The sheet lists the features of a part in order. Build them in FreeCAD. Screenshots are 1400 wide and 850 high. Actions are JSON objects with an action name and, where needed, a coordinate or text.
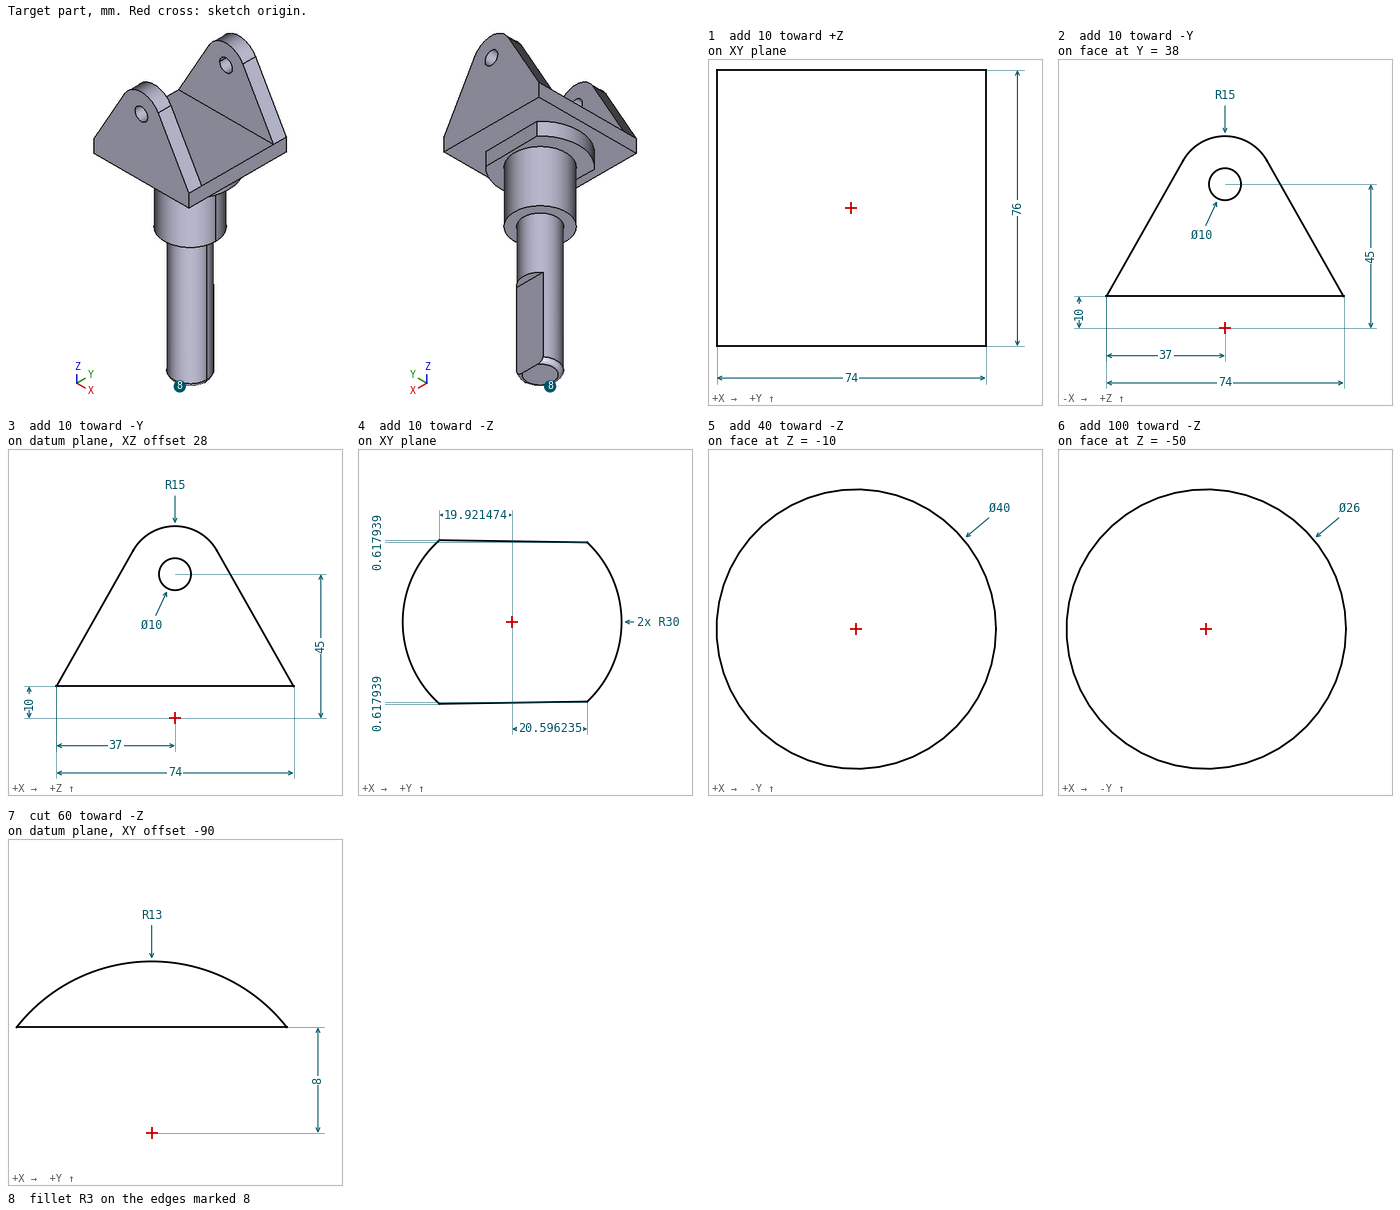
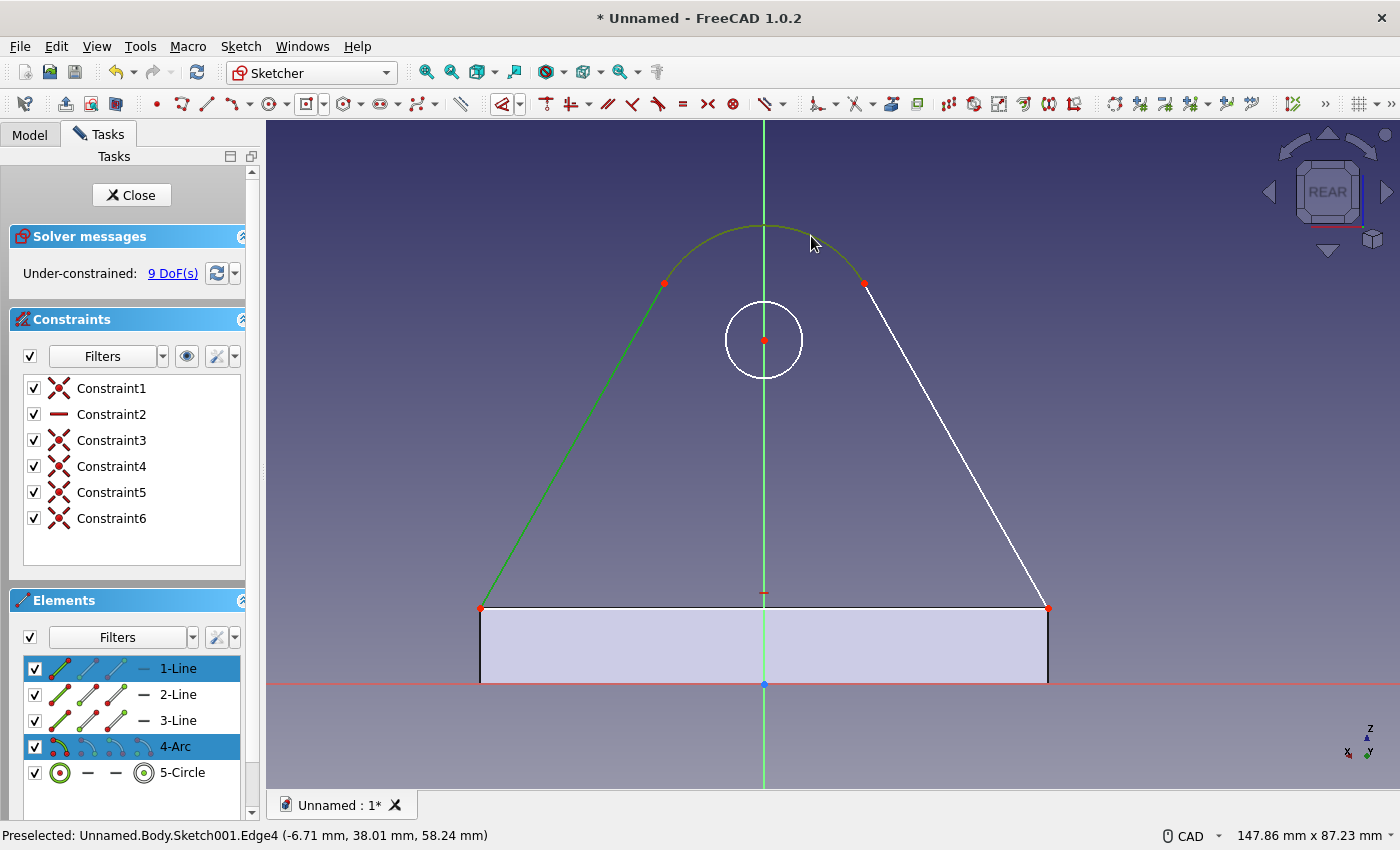
{"action": "left_click", "coordinate": [658, 104]}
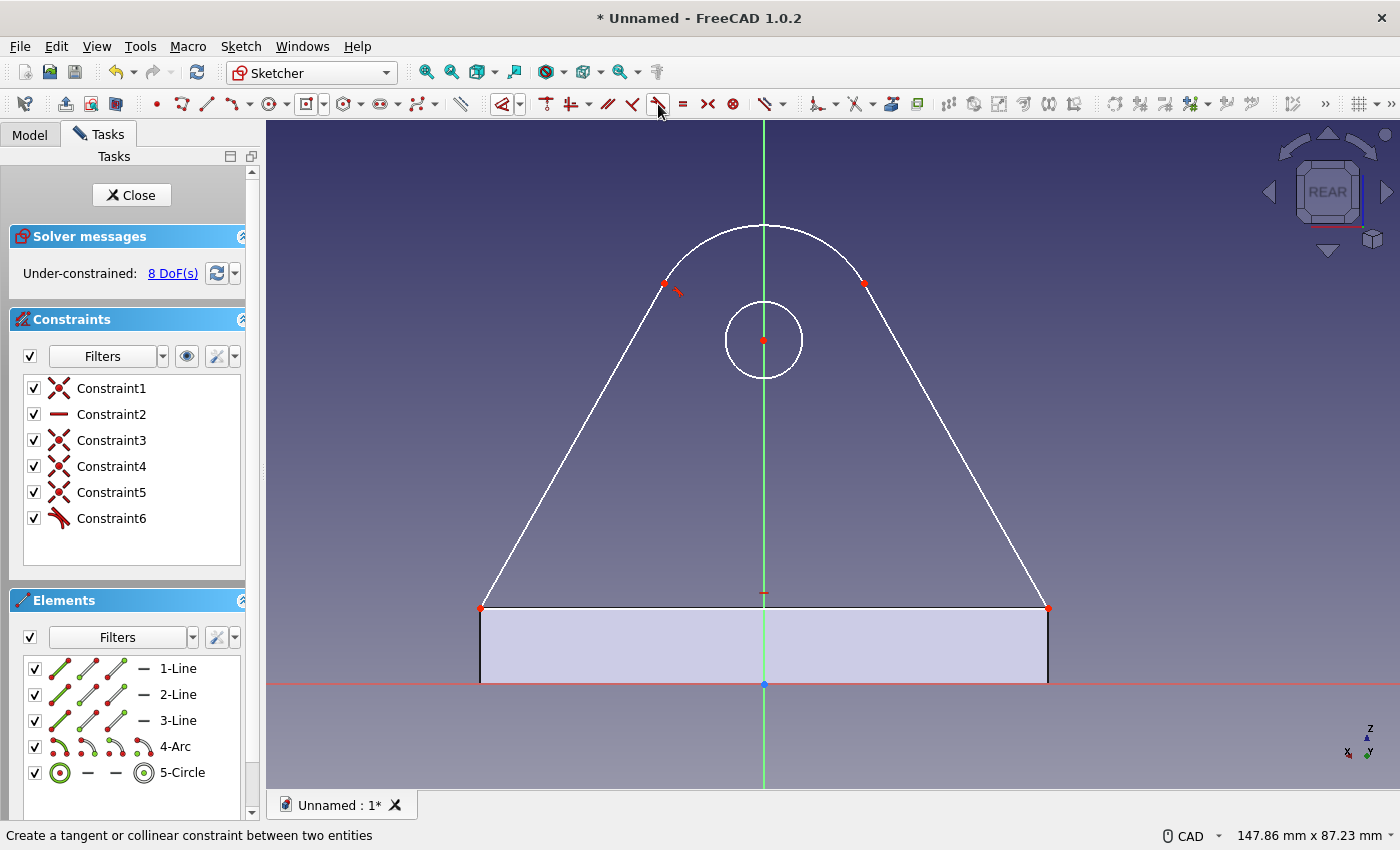
{"action": "left_click", "coordinate": [993, 511]}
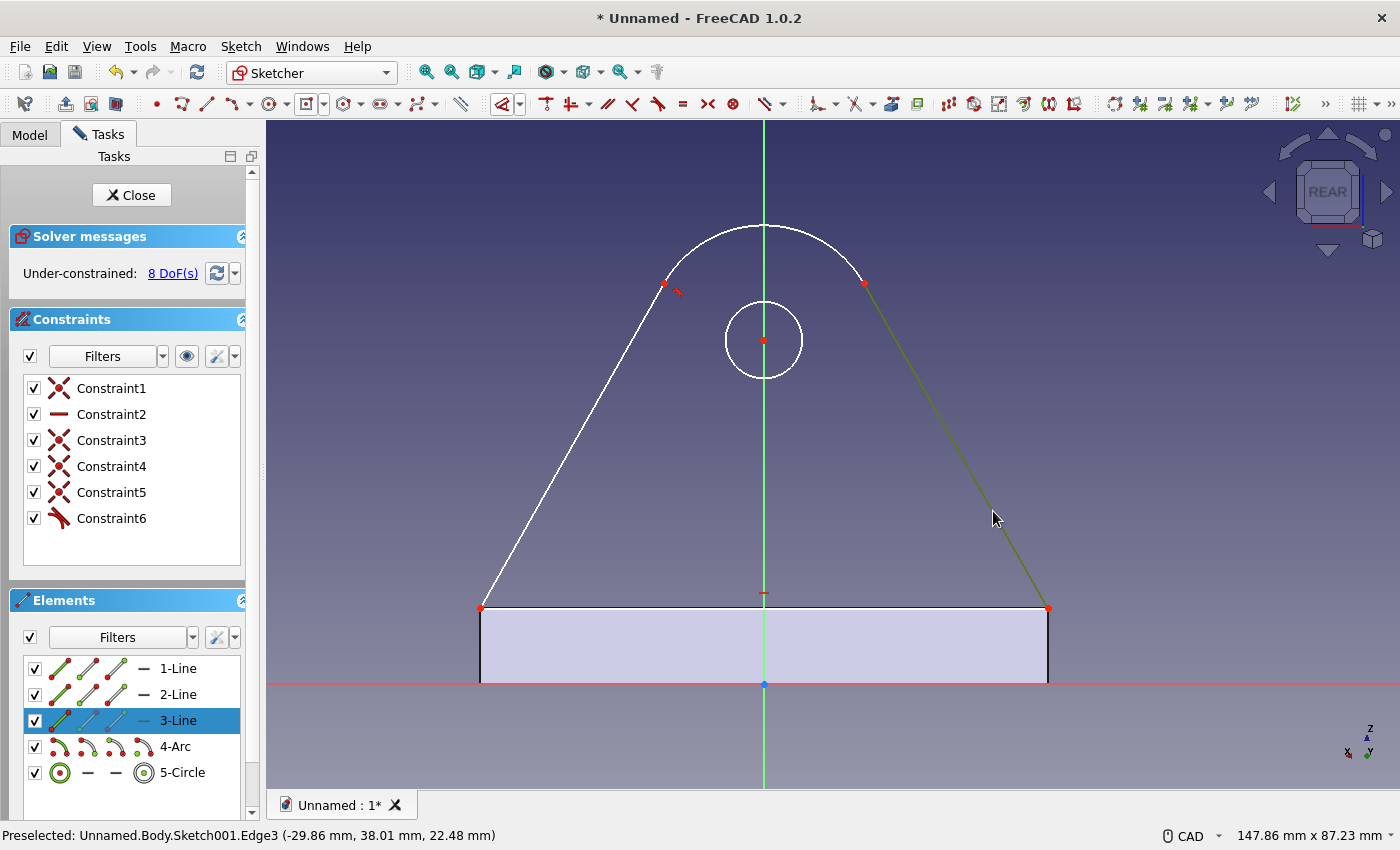
{"action": "left_click", "coordinate": [811, 236]}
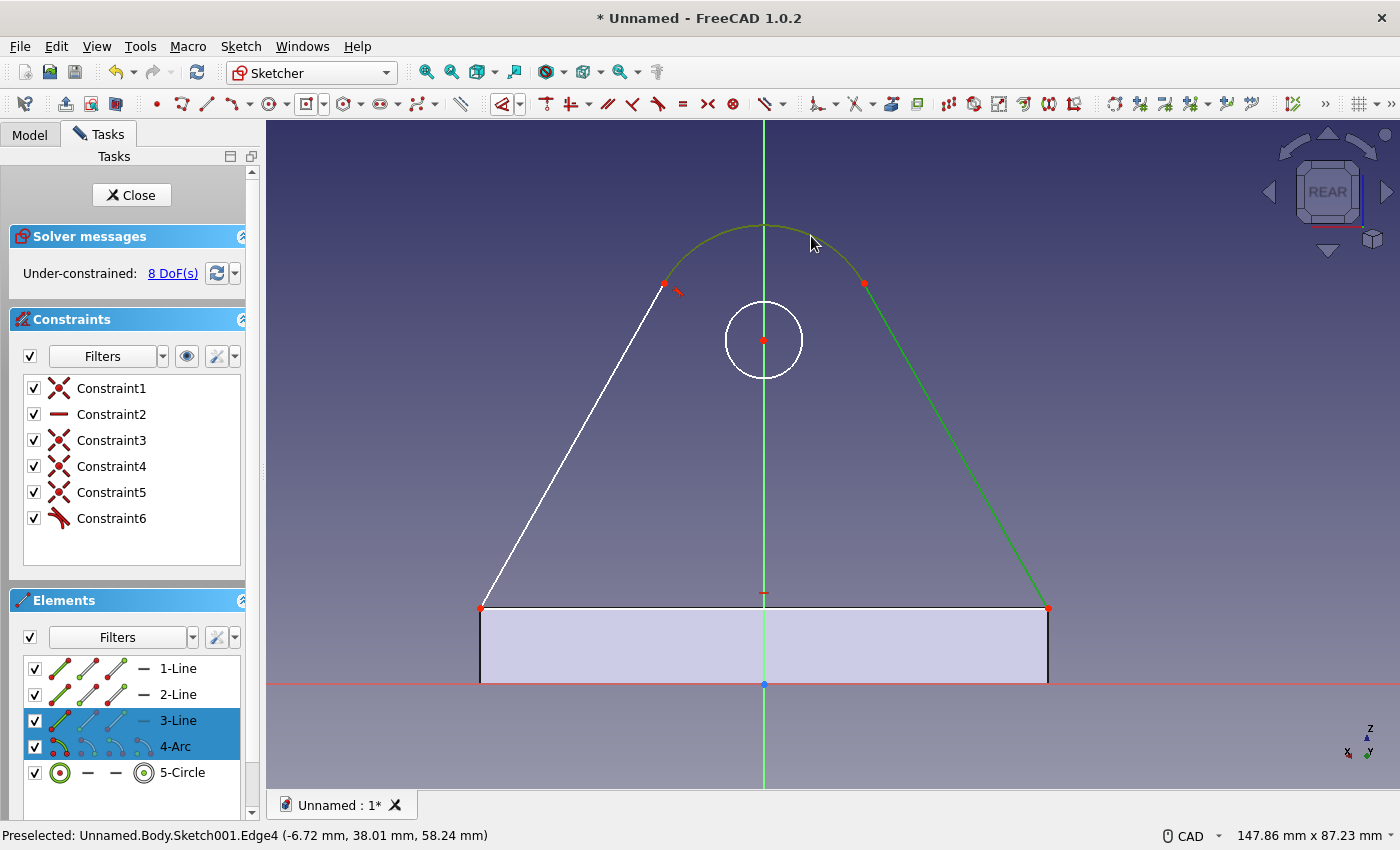
{"action": "left_click", "coordinate": [658, 104]}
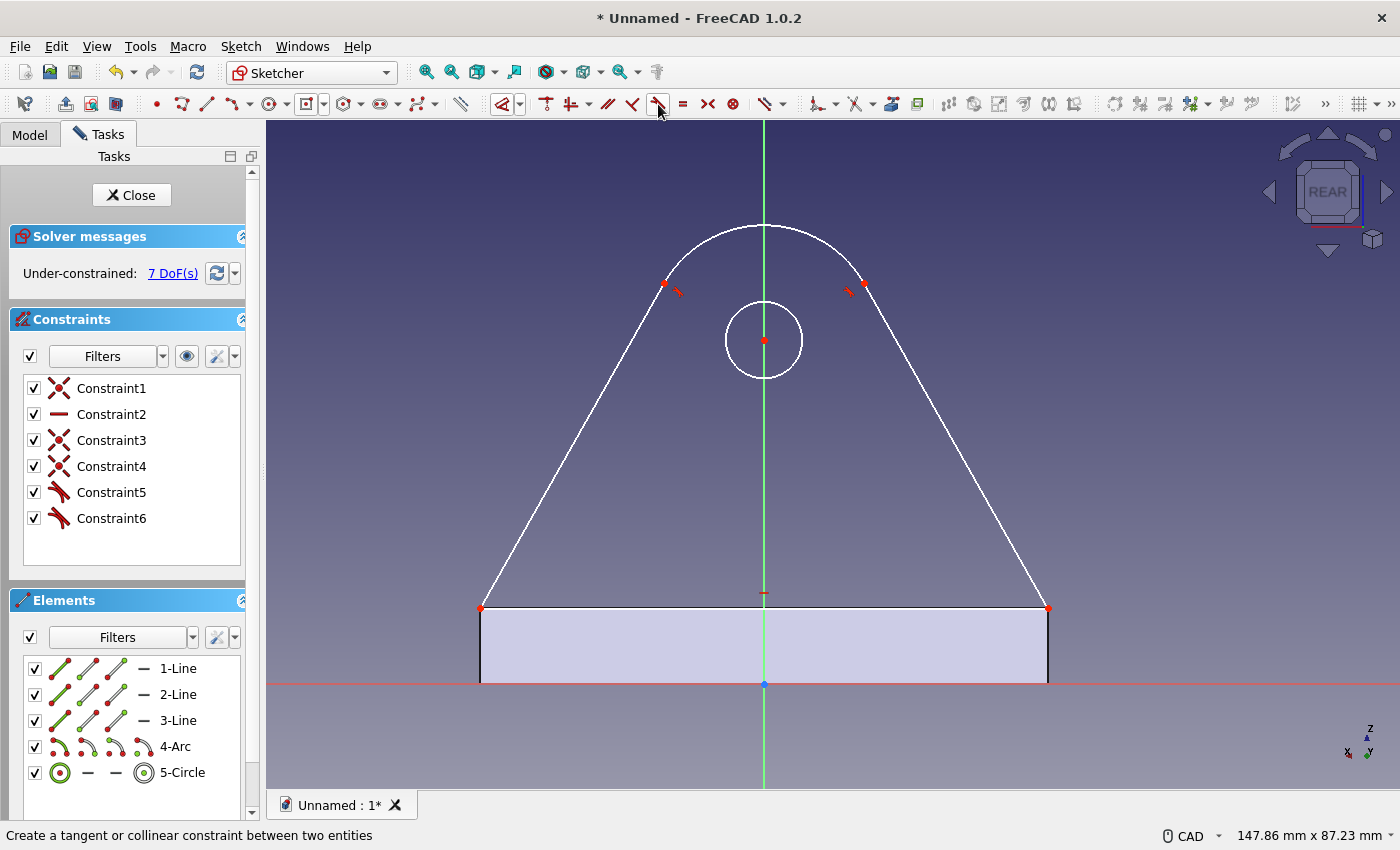
{"action": "left_click", "coordinate": [764, 340]}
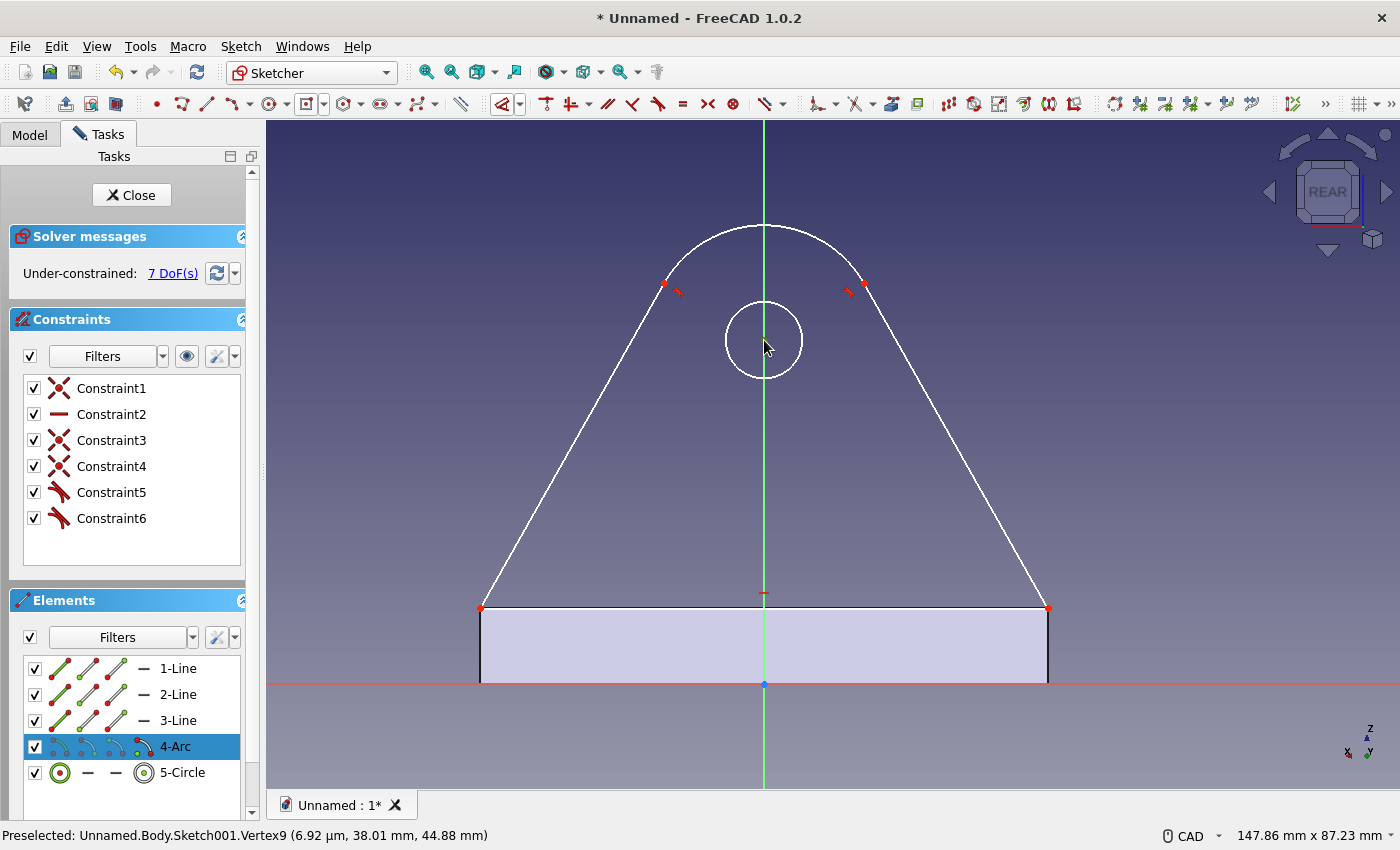
{"action": "left_click", "coordinate": [764, 717]}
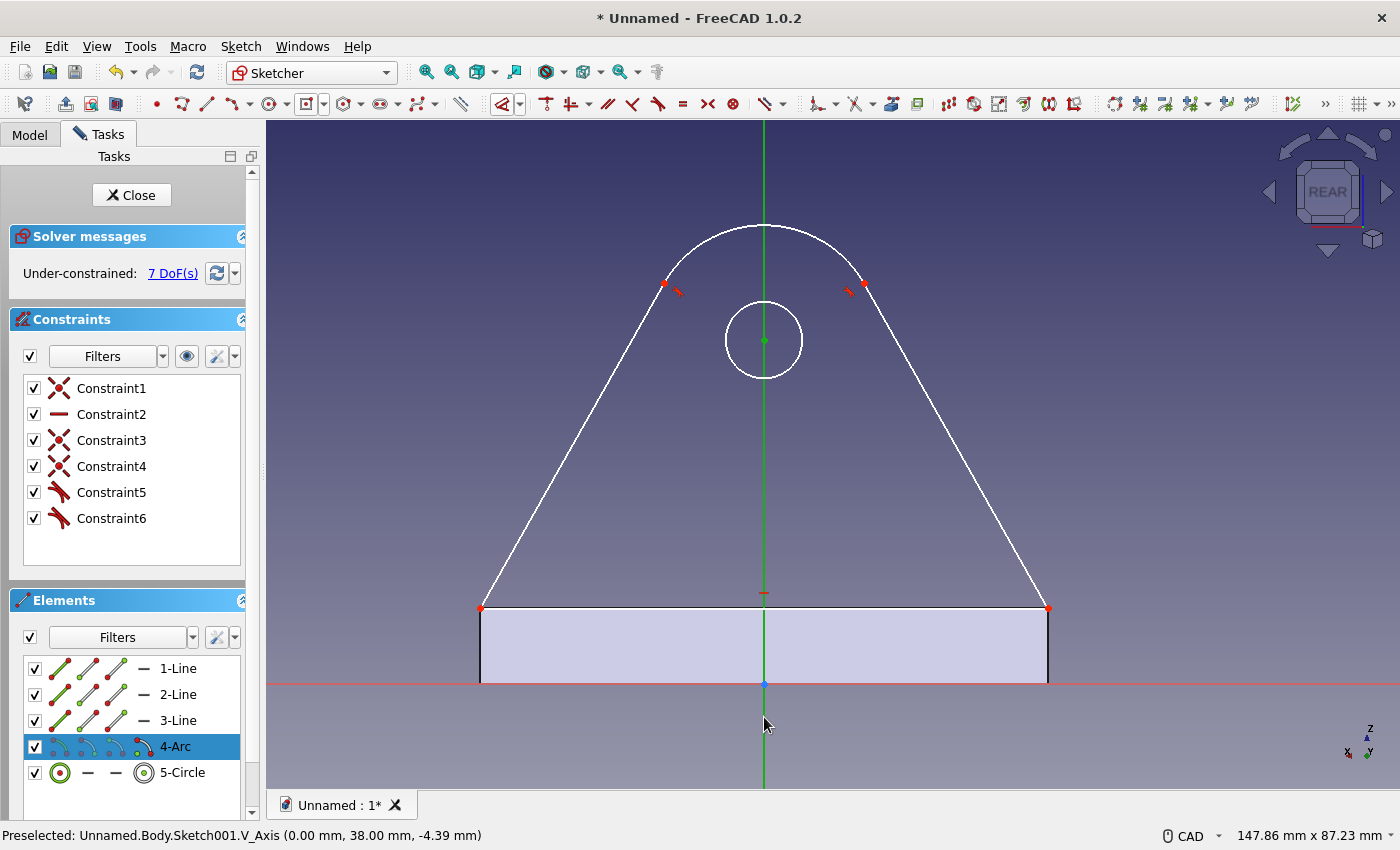
{"action": "key", "text": "c"}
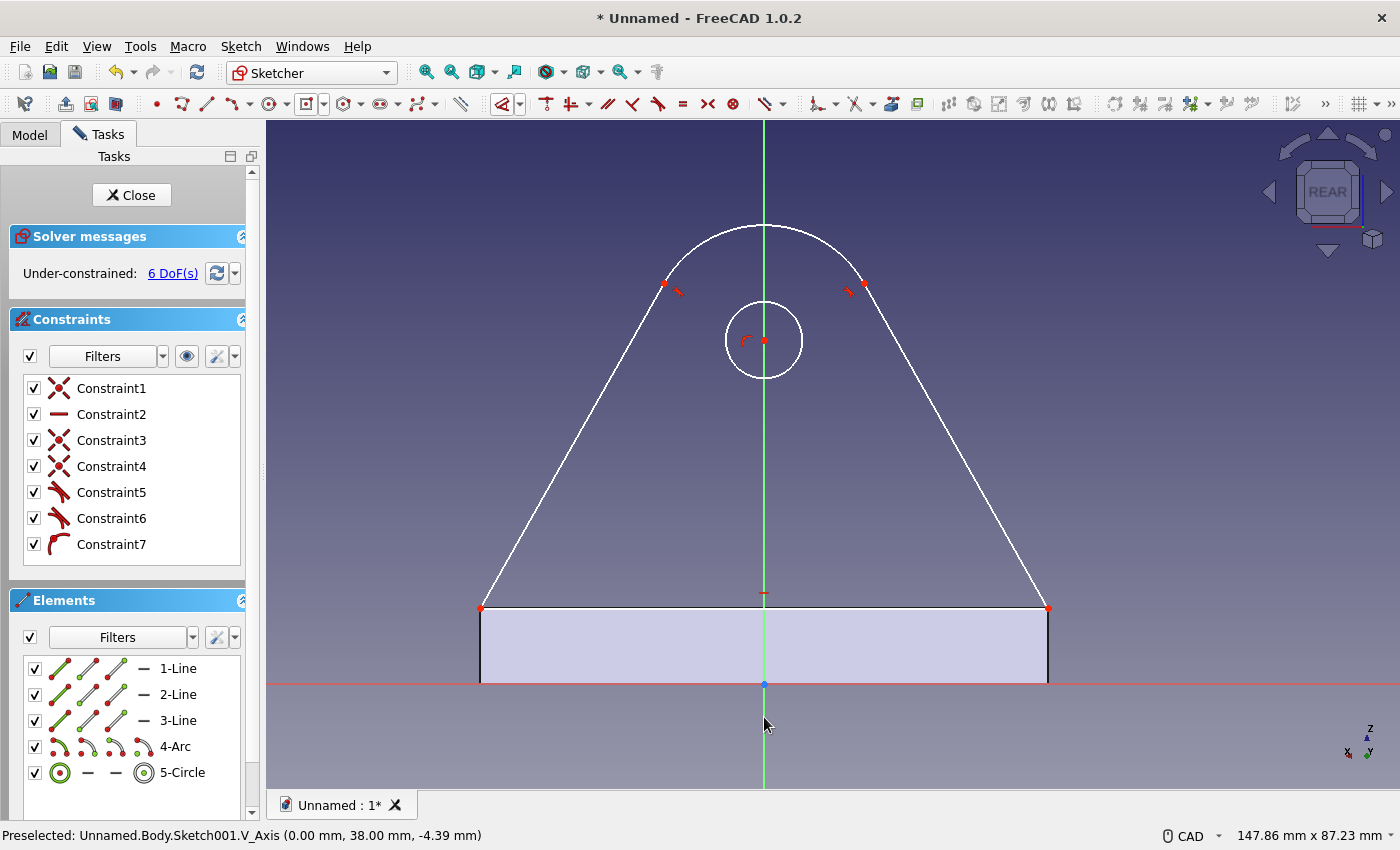
{"action": "left_click", "coordinate": [811, 235]}